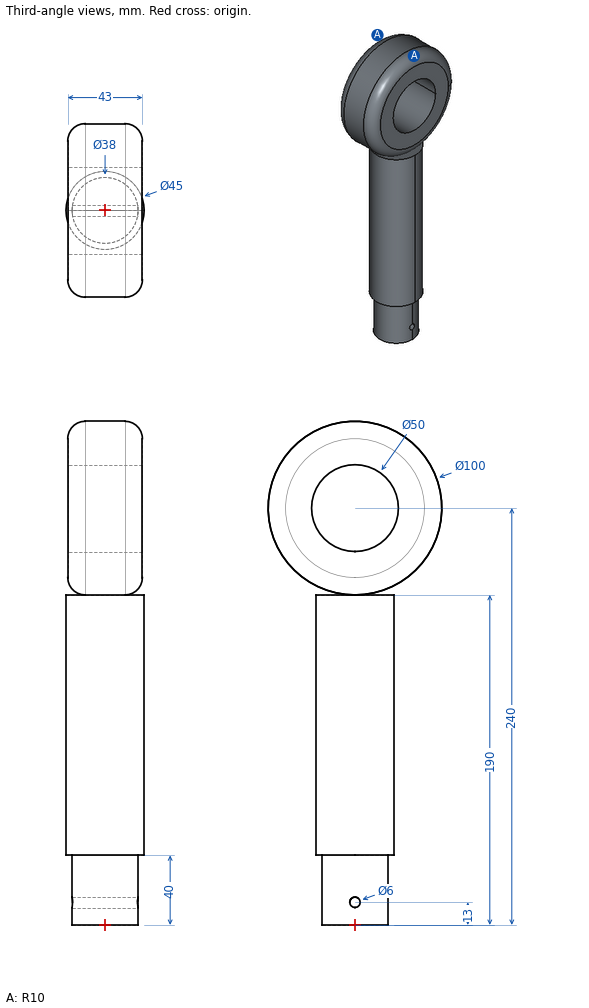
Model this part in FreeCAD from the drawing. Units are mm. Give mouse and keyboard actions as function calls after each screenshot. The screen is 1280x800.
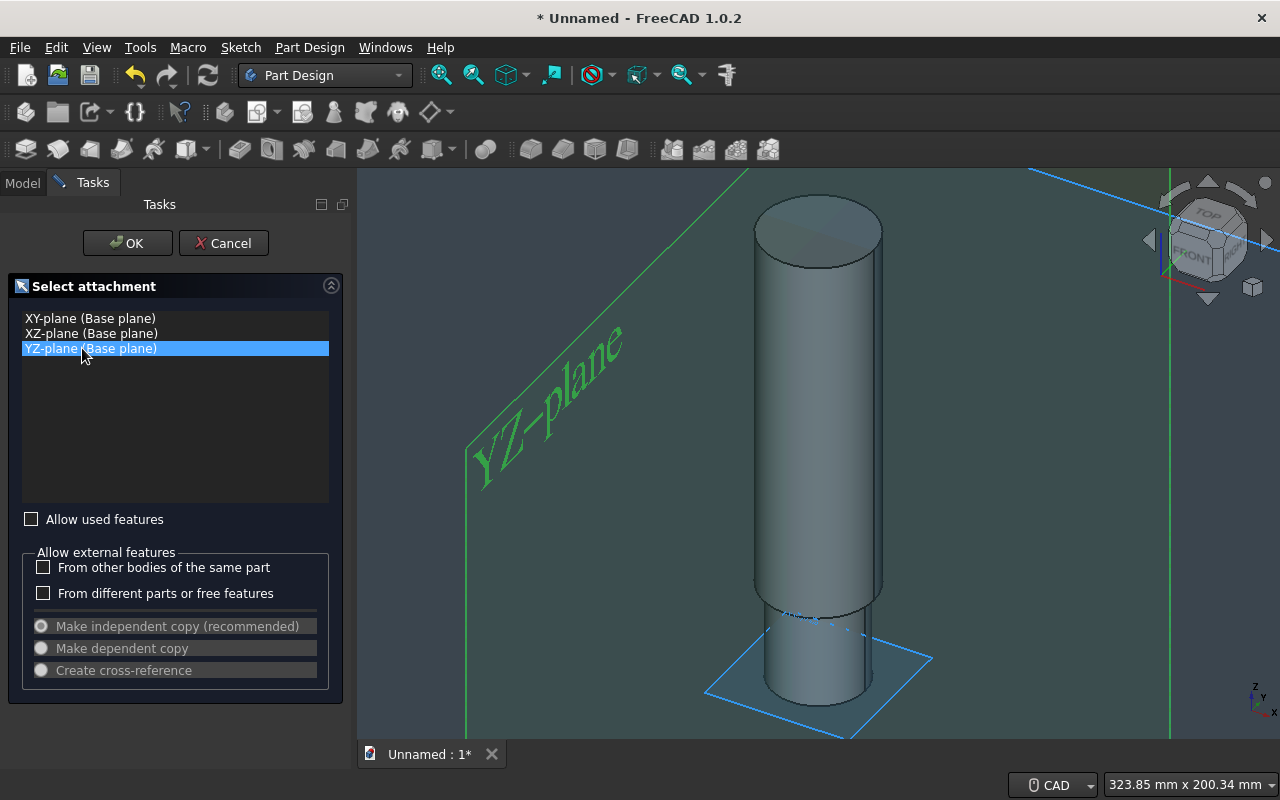
click(128, 243)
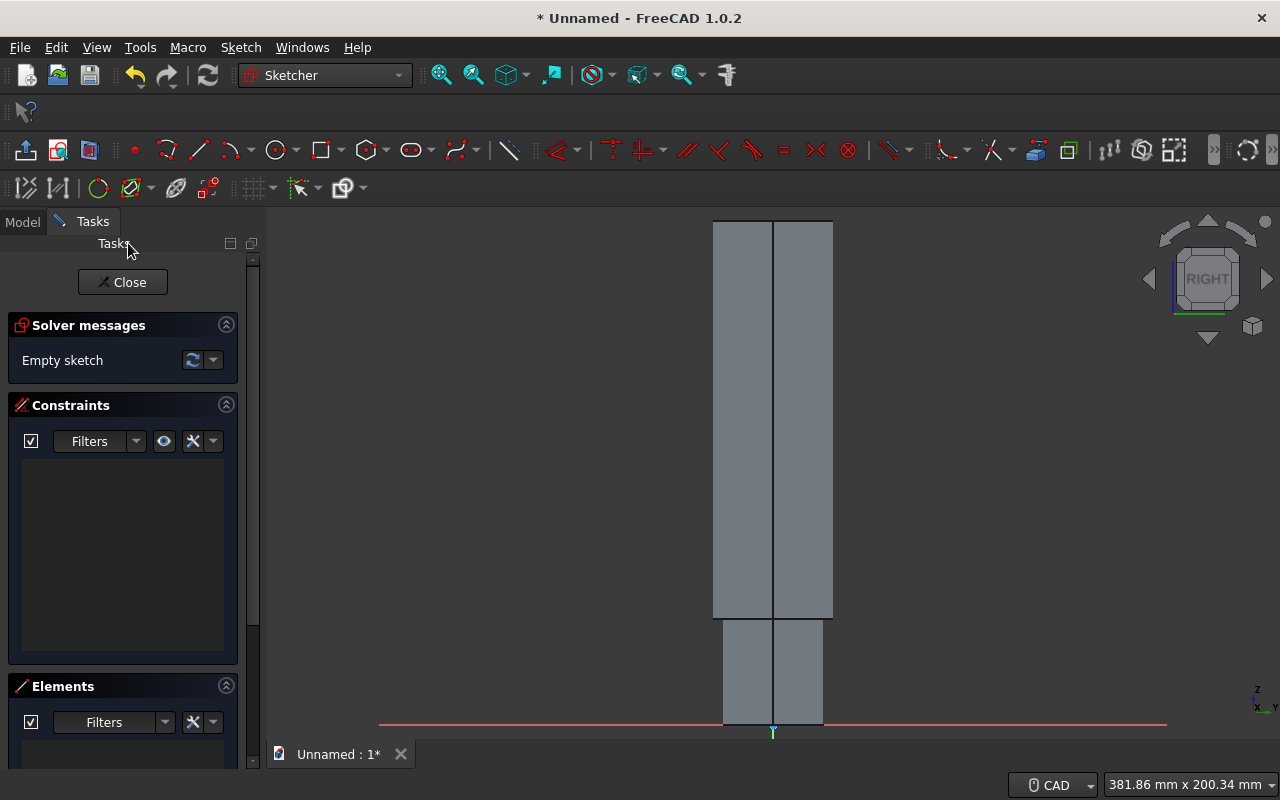
click(90, 150)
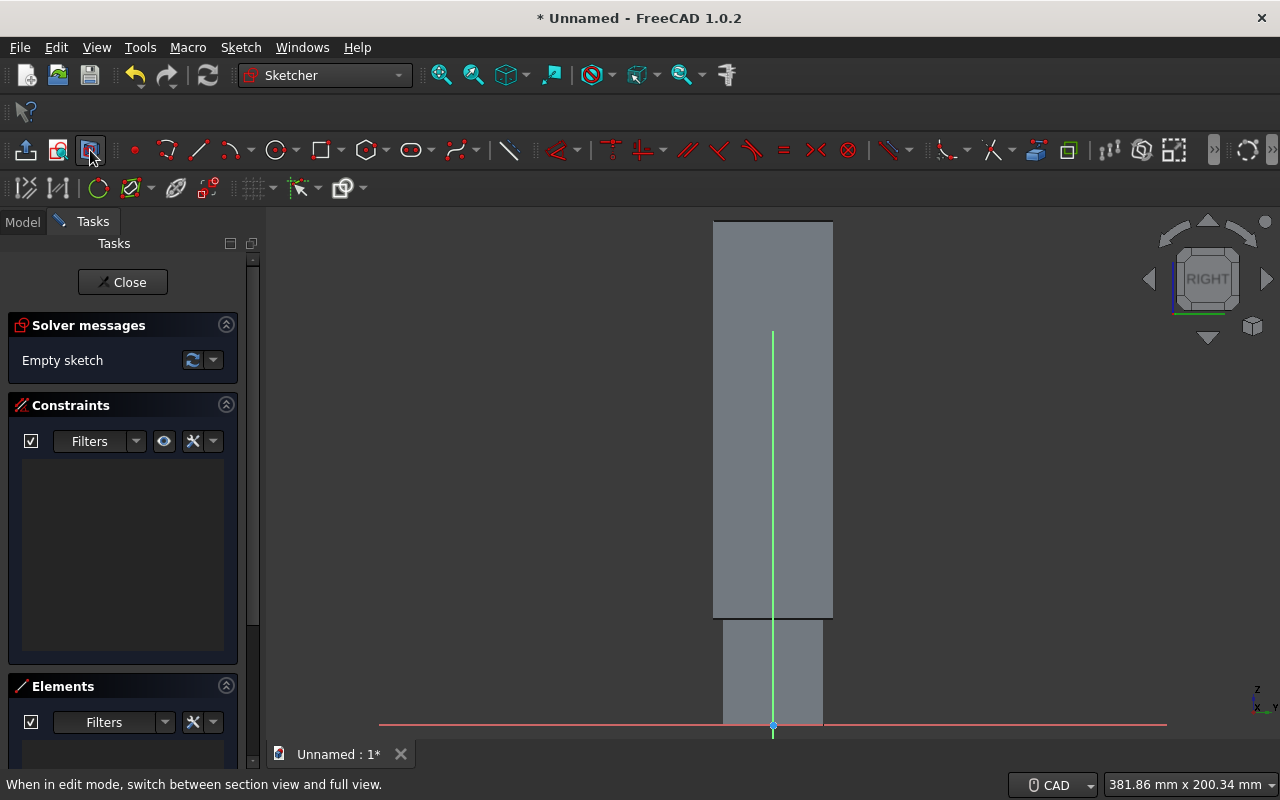
scroll(777, 702, up, 15)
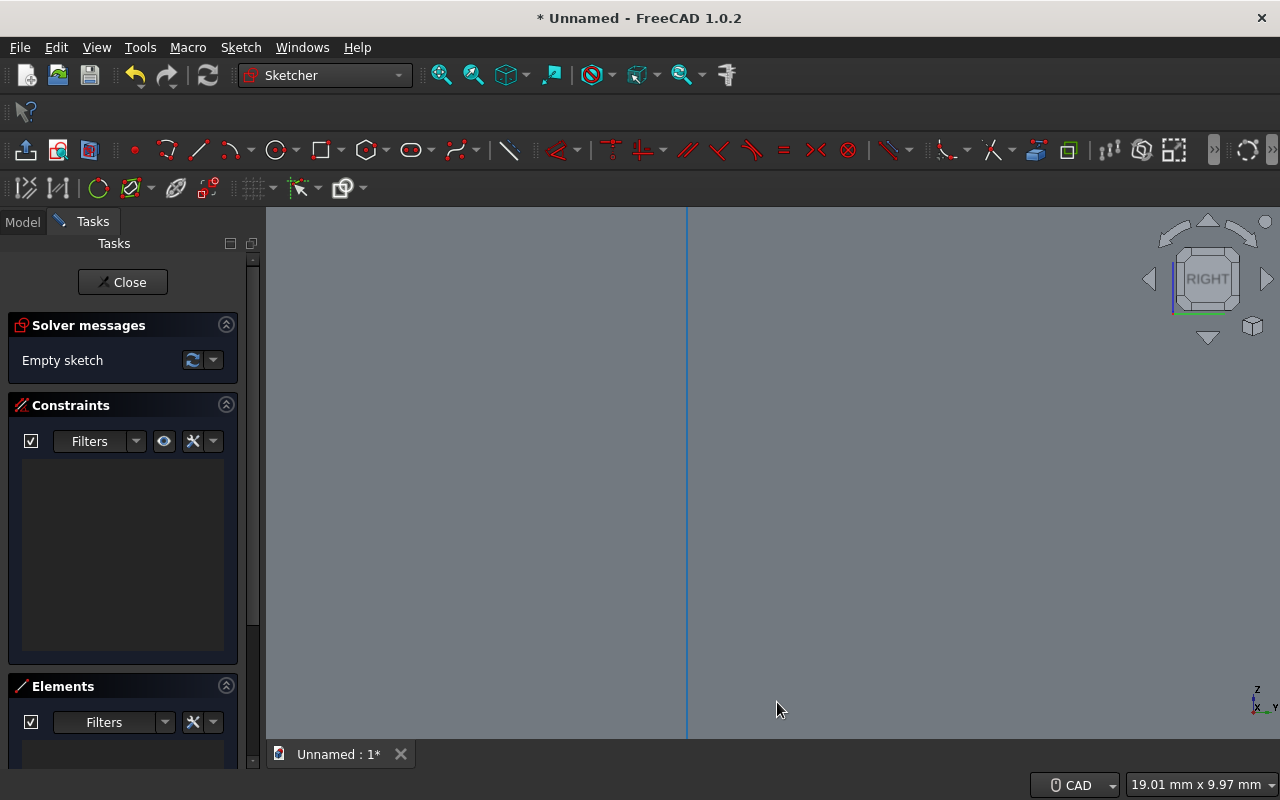
click(276, 150)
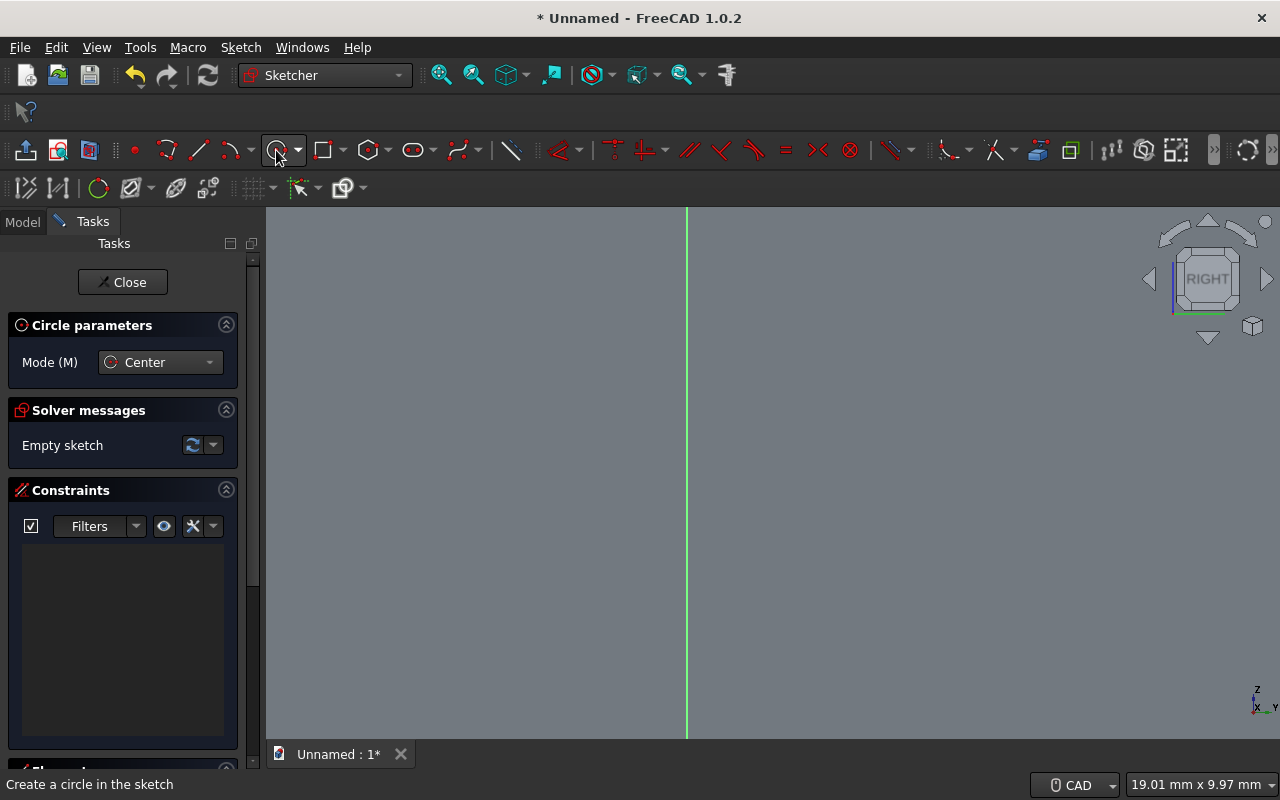
click(687, 458)
move(800, 345)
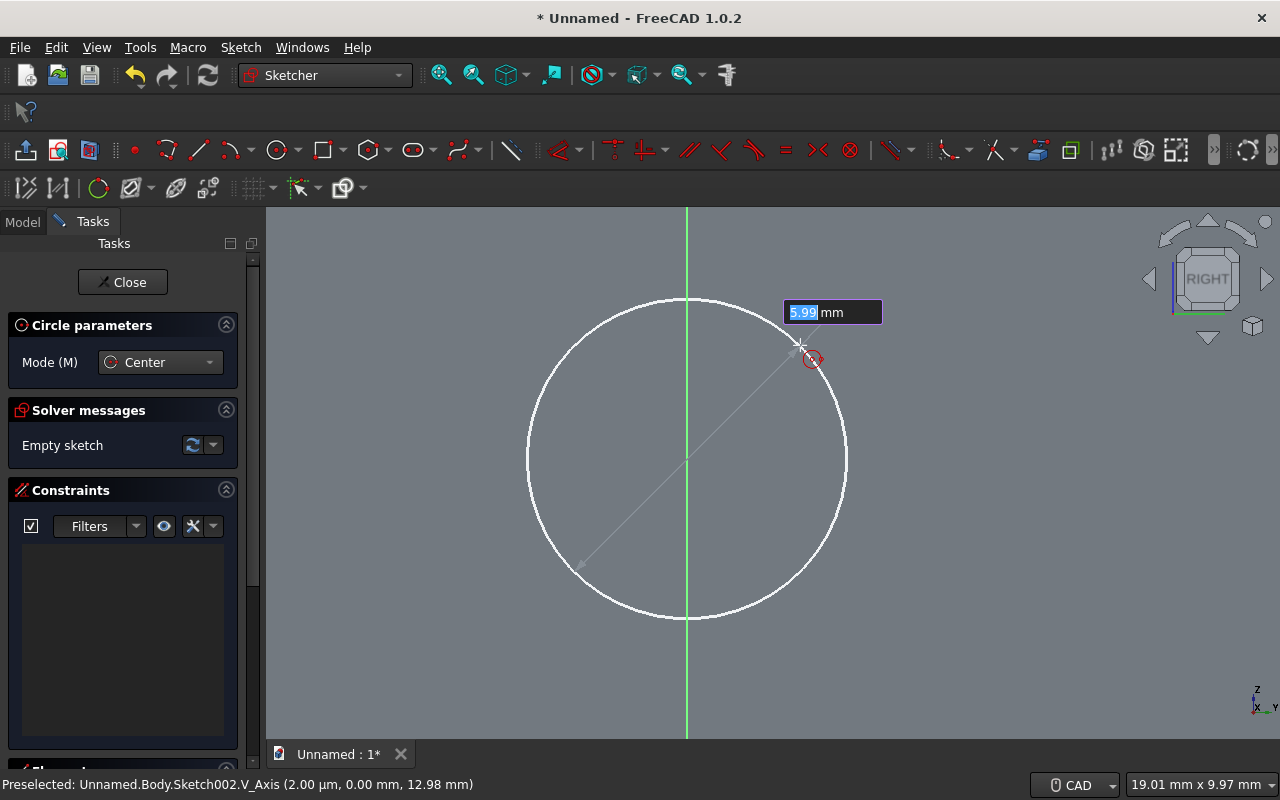
text(6)
key(Return)
key(Escape)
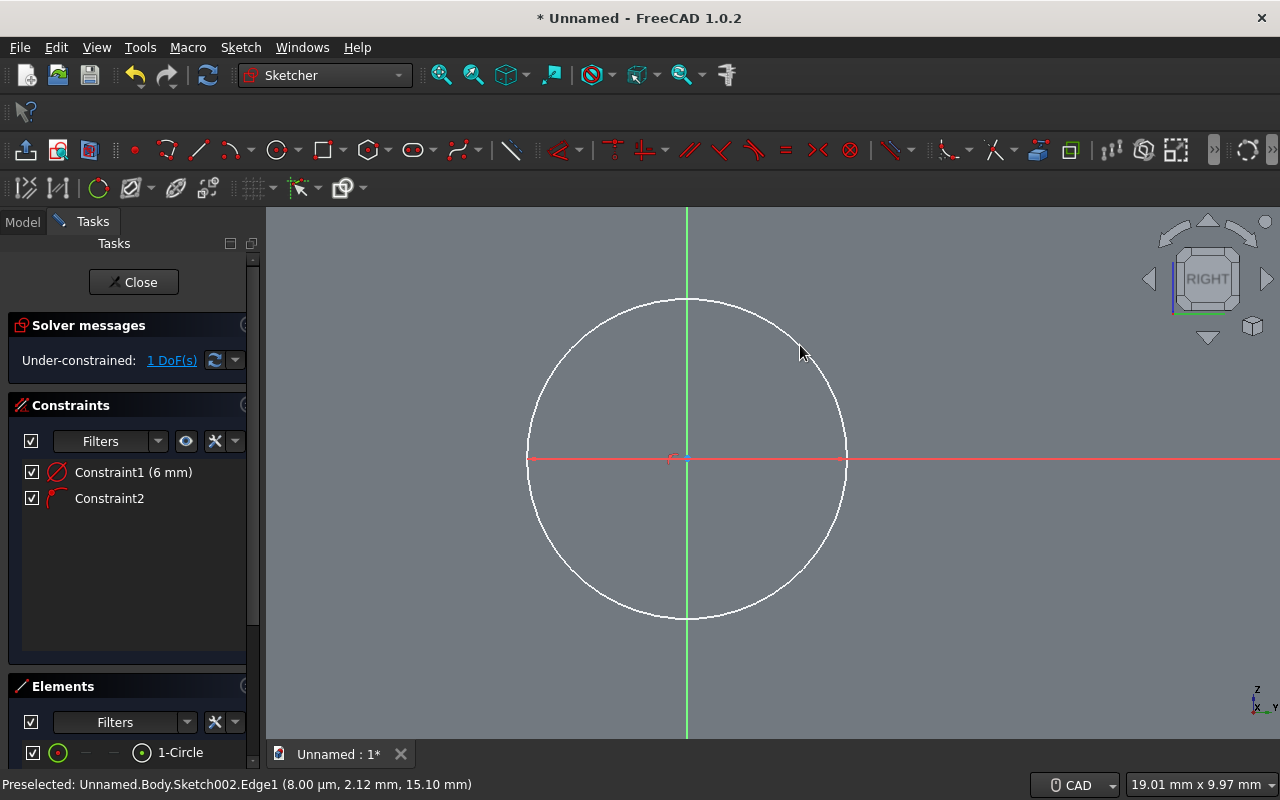
key(d)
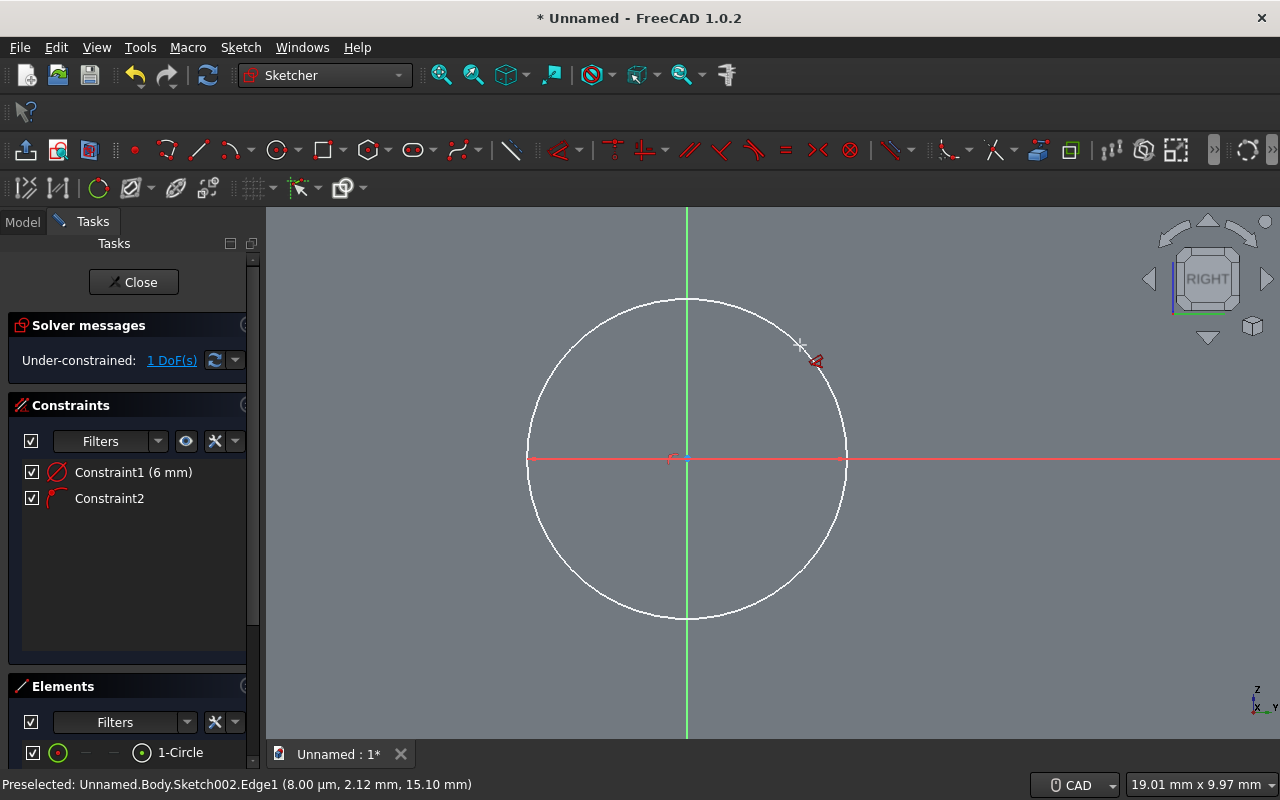
click(687, 459)
click(721, 585)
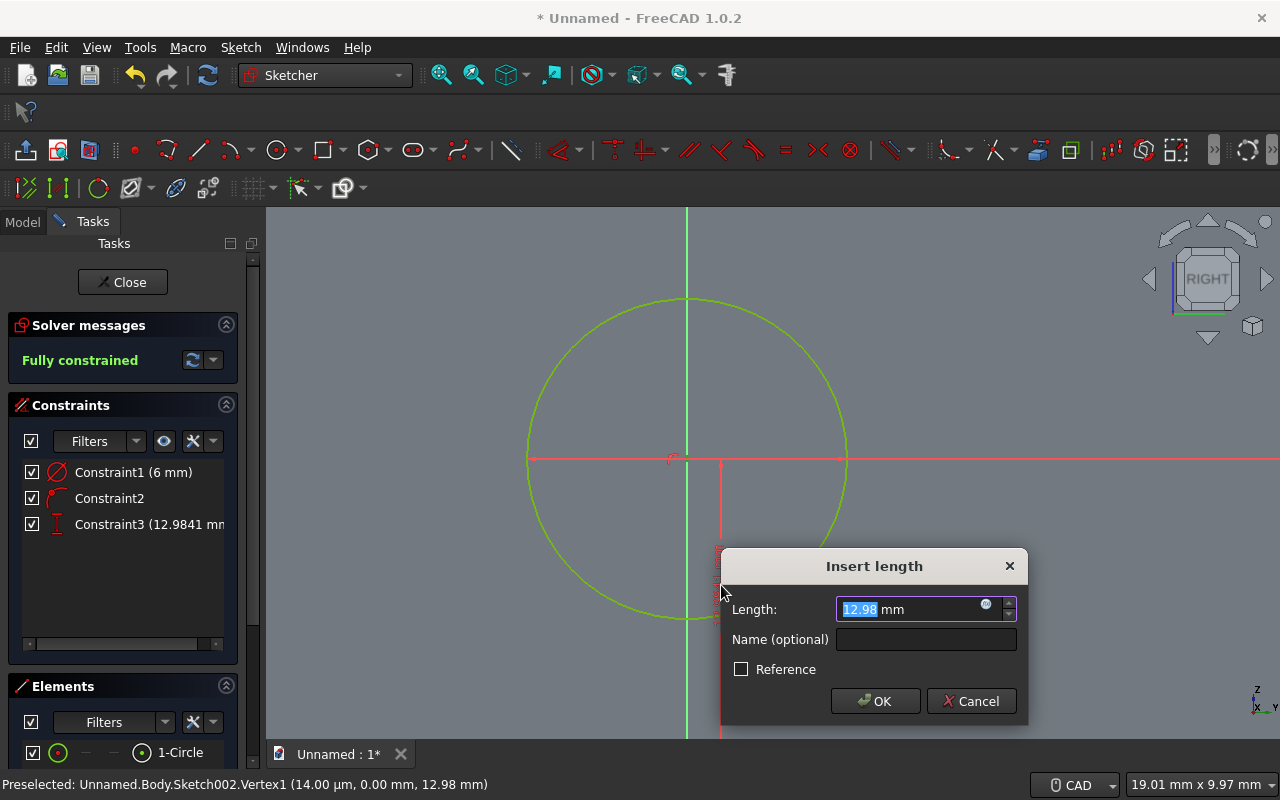
text(13)
key(Return)
key(Escape)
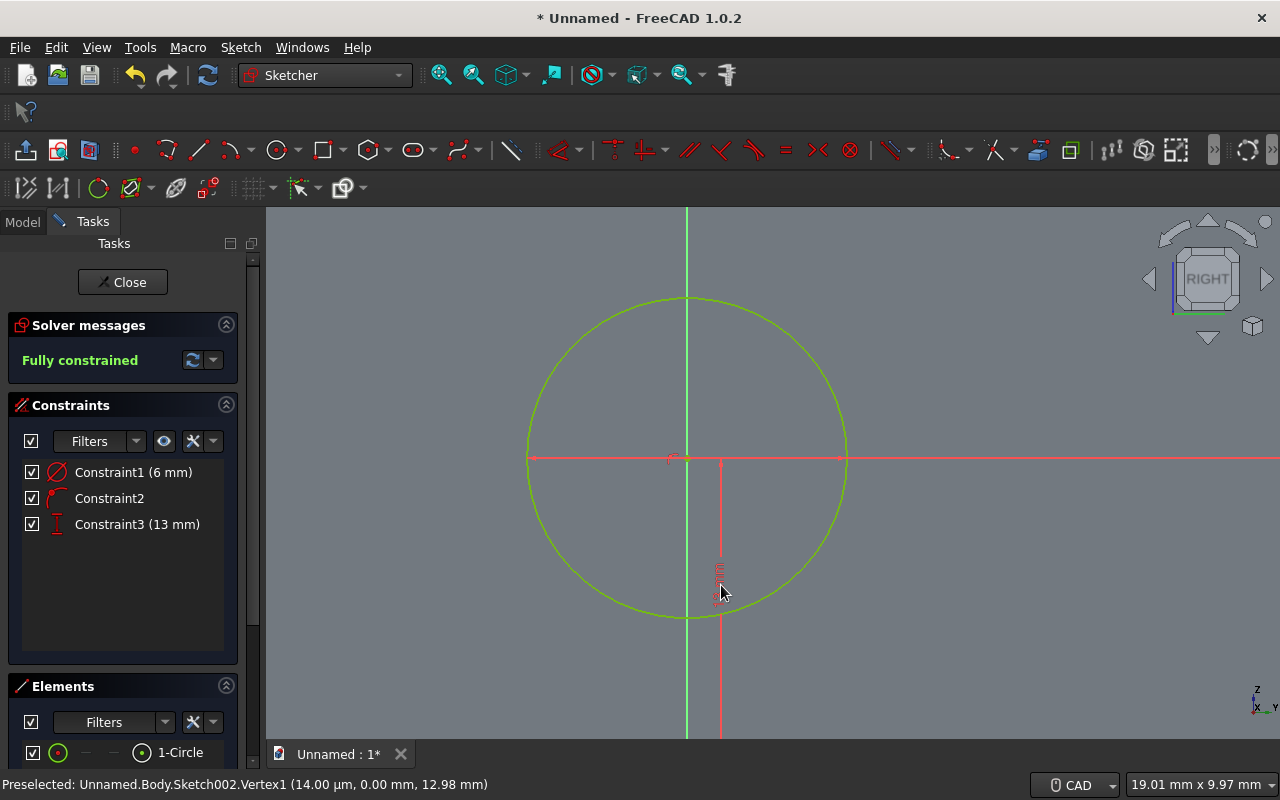
click(123, 282)